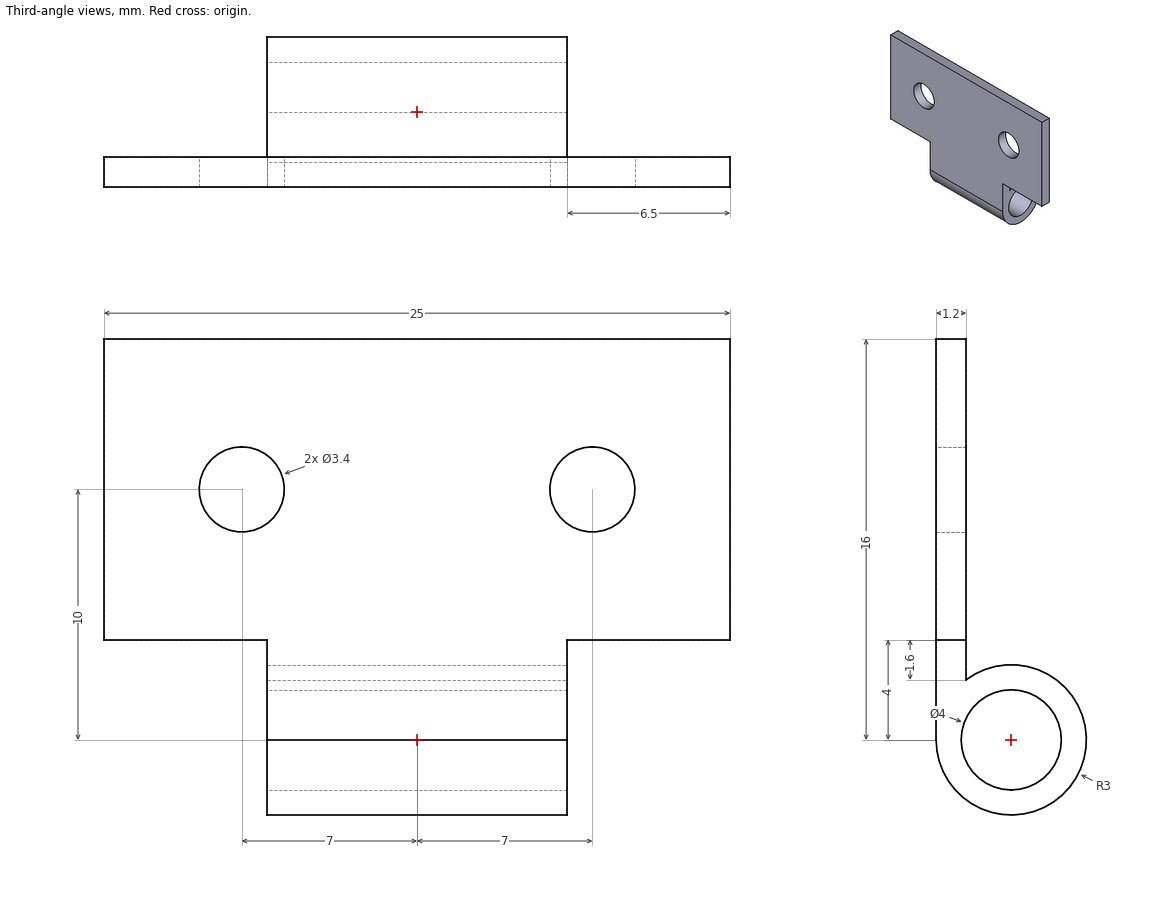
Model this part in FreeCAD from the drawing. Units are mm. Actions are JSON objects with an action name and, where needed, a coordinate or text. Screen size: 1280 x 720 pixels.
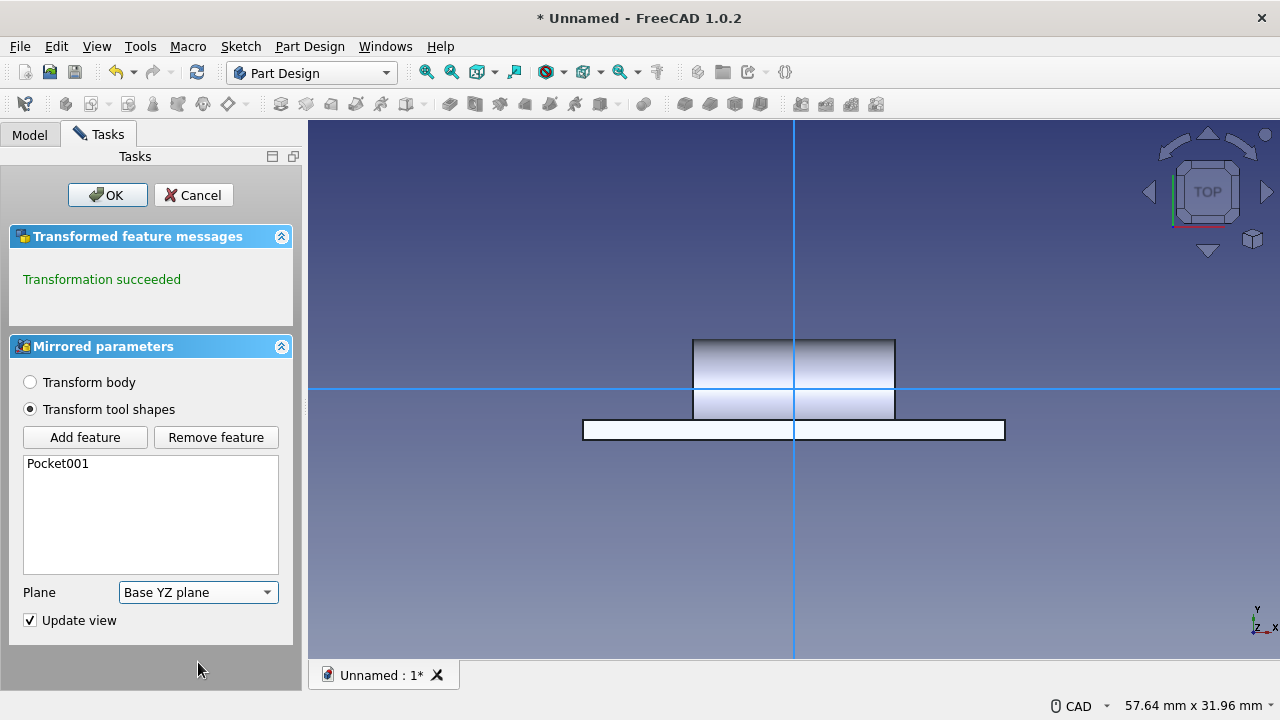
{"action": "left_click", "coordinate": [108, 195]}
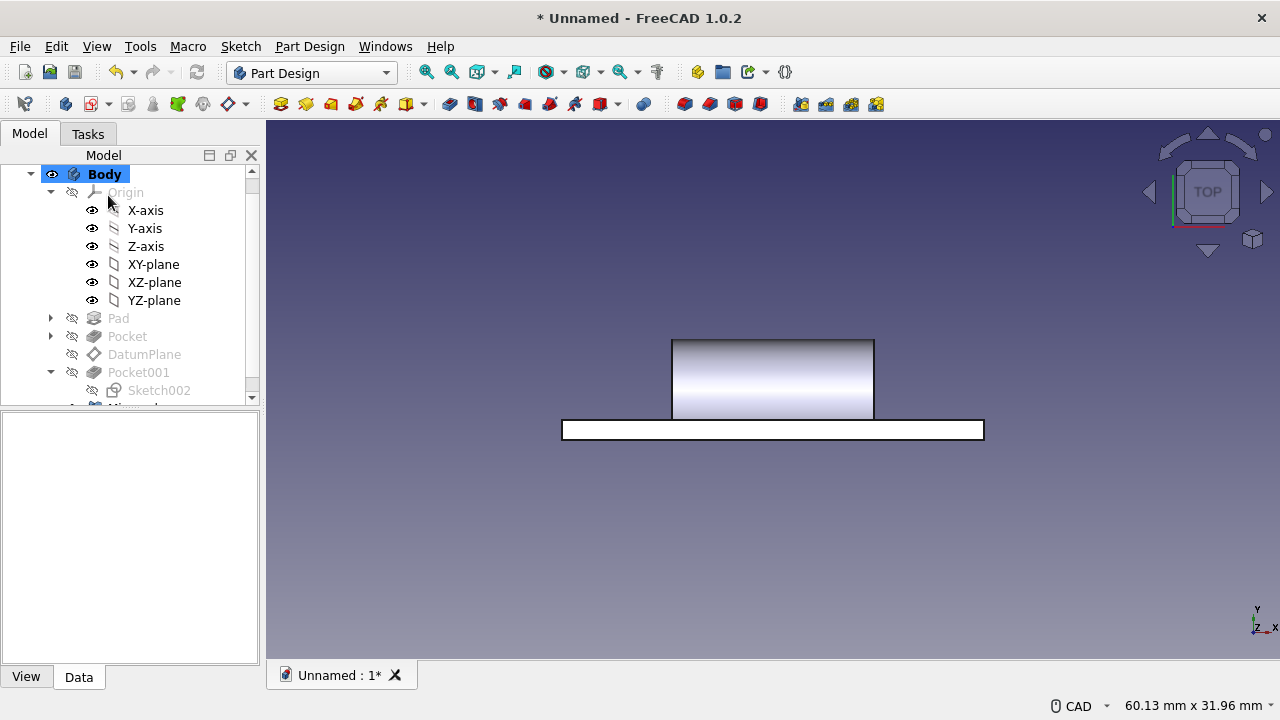
{"action": "key", "text": "0"}